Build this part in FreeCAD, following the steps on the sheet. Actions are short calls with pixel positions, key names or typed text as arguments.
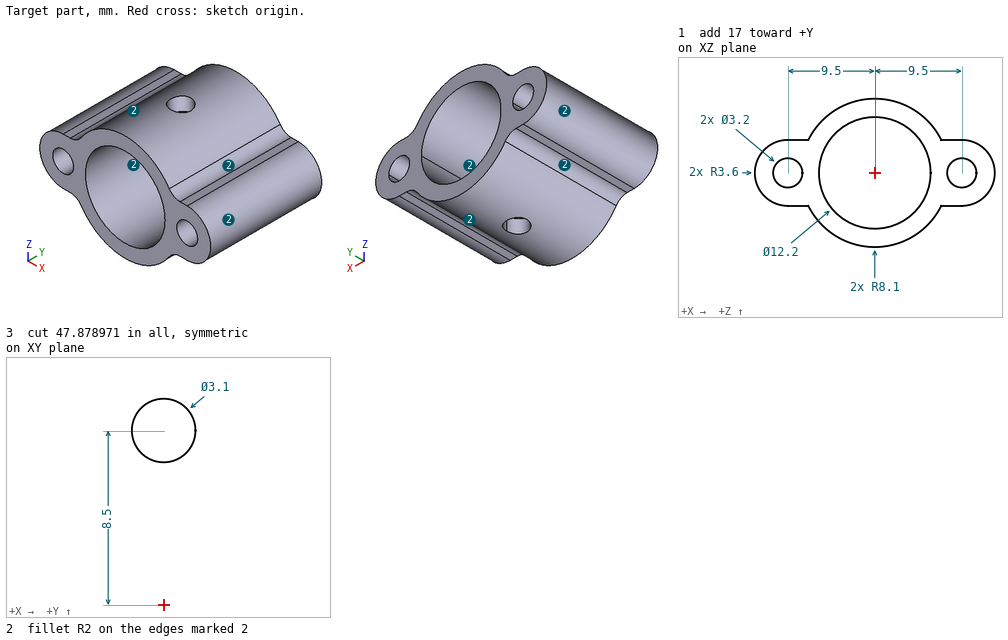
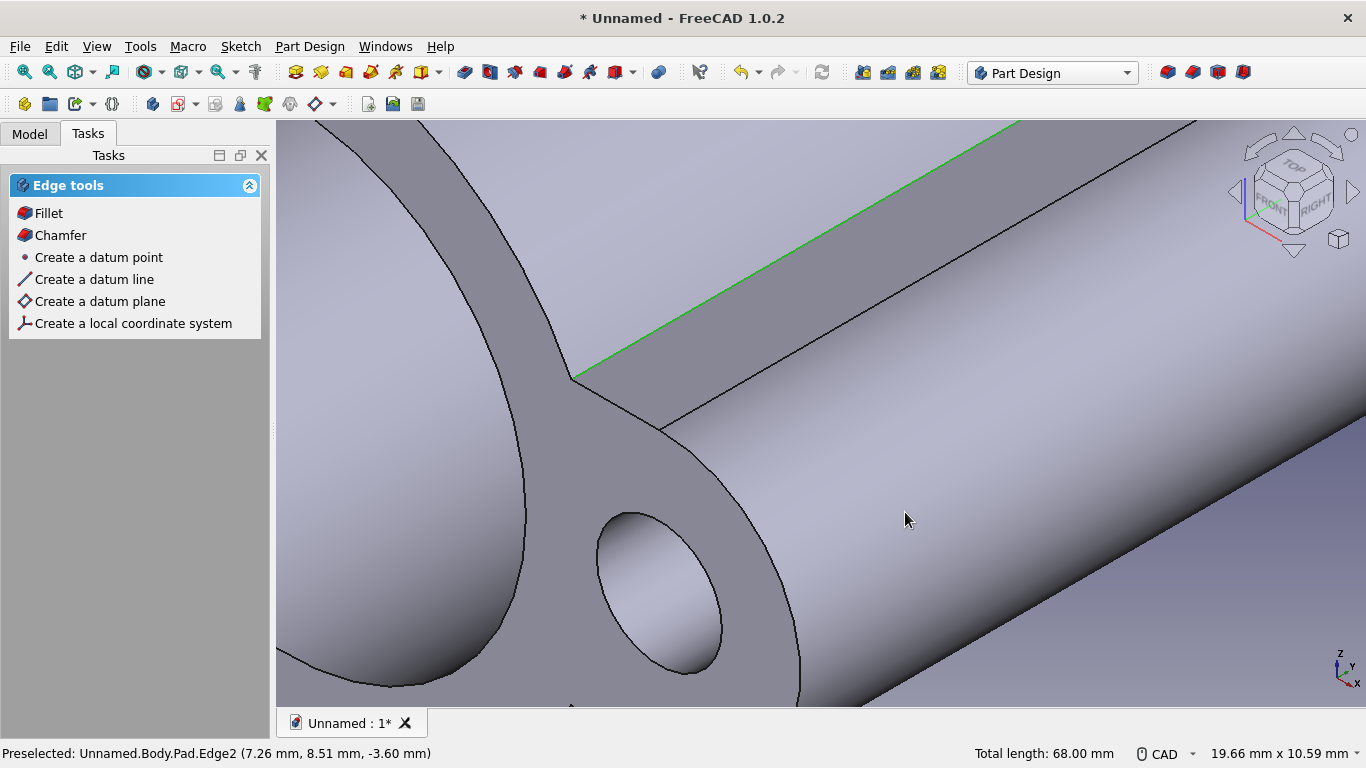
click(1168, 72)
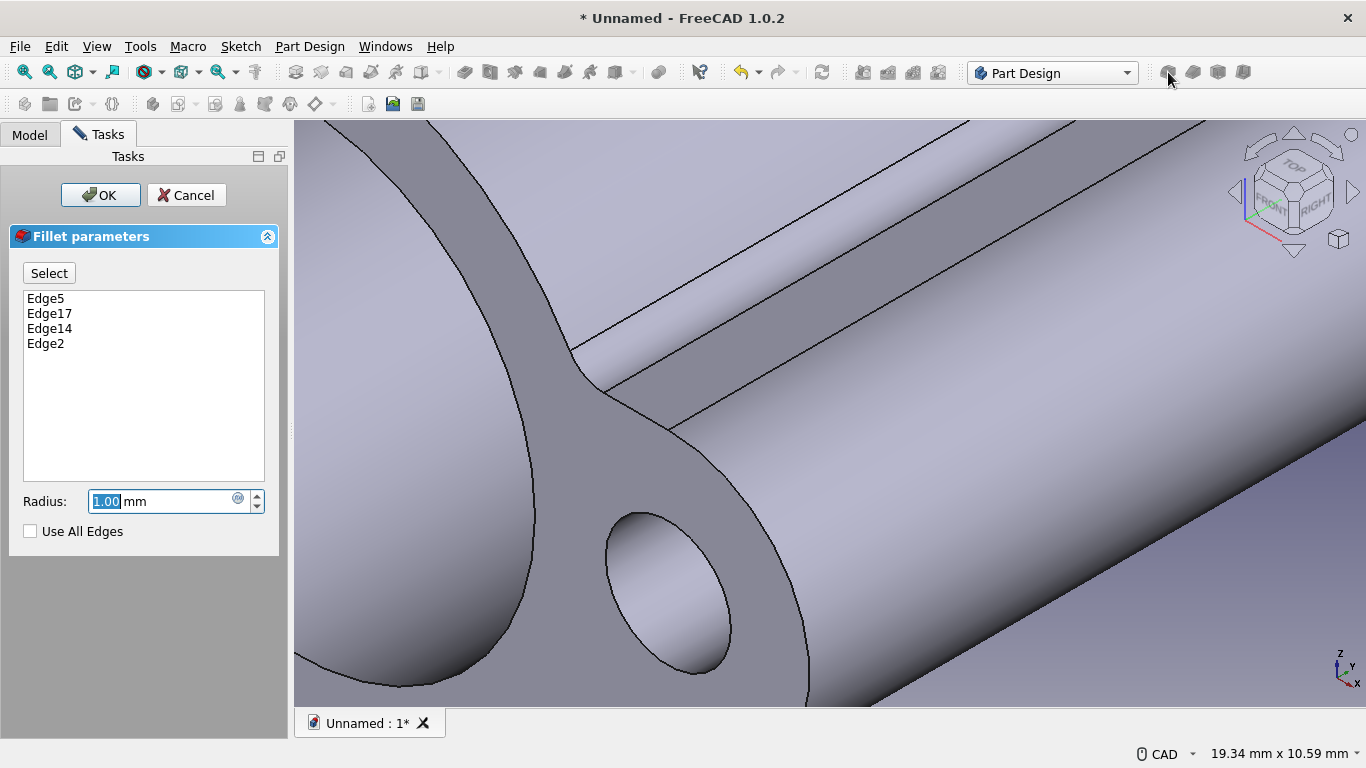
text(2)
key(Tab)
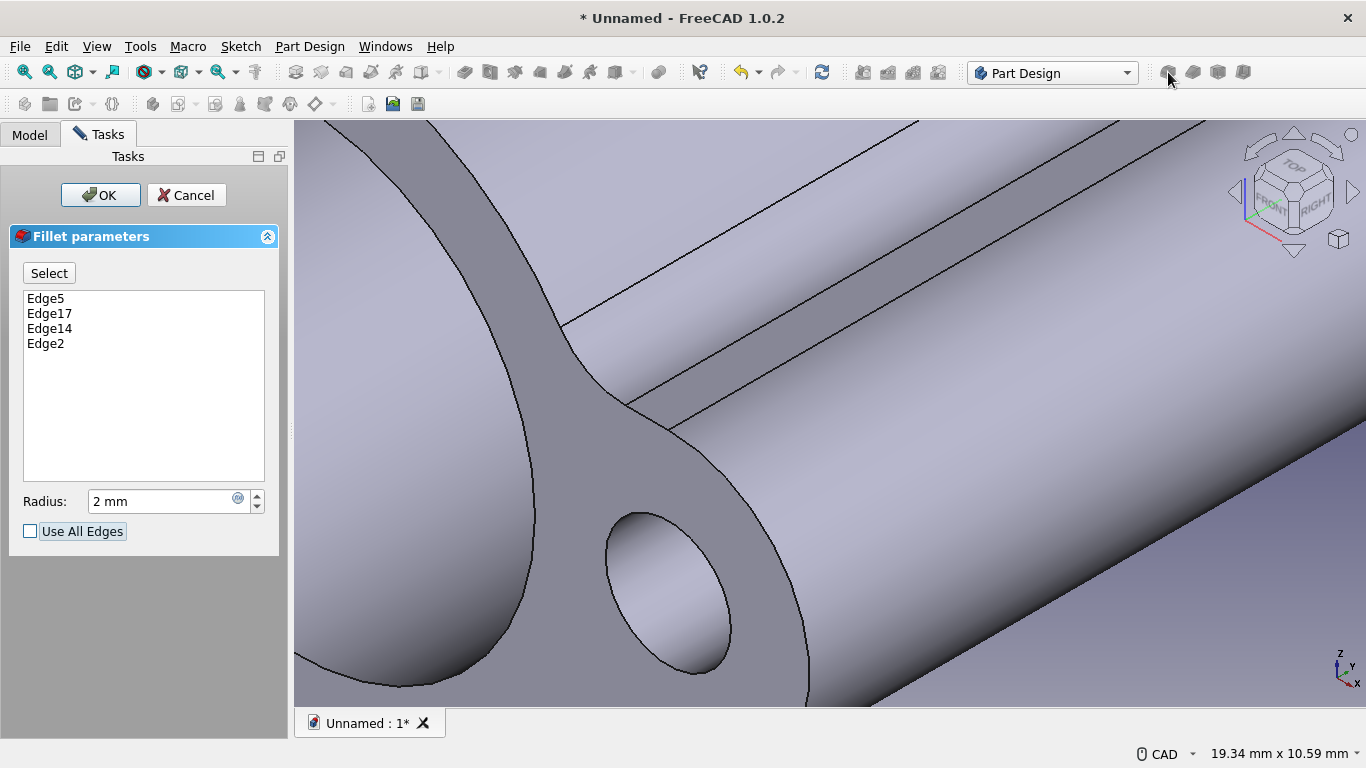
click(101, 195)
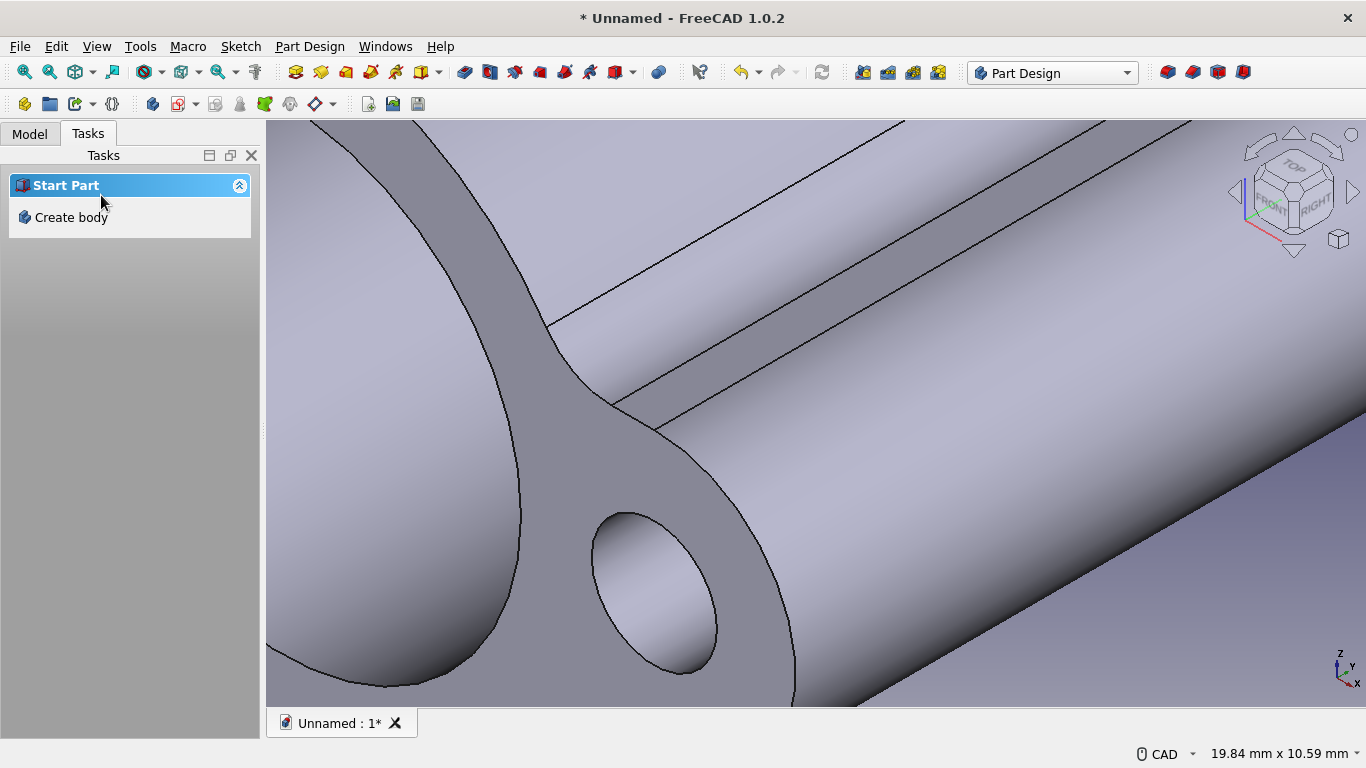
key(v)
key(f)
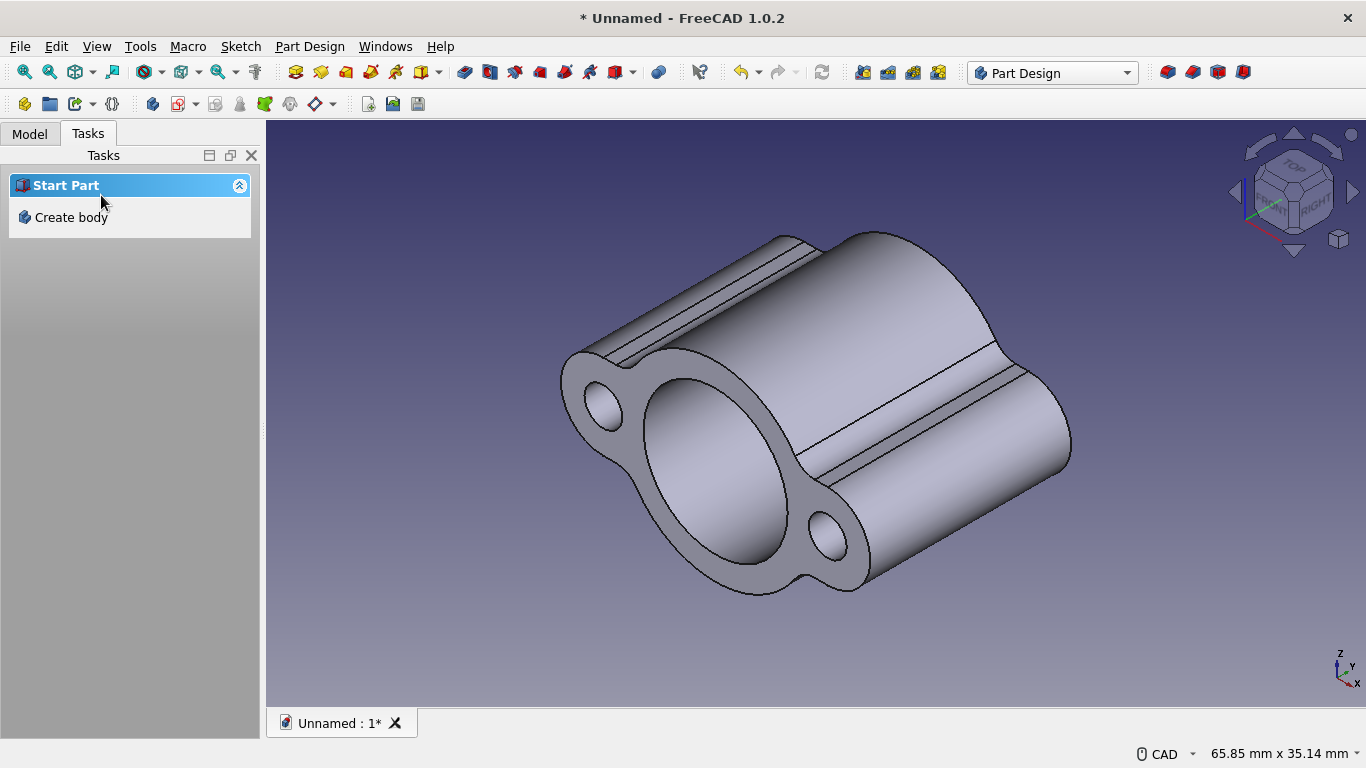
click(178, 104)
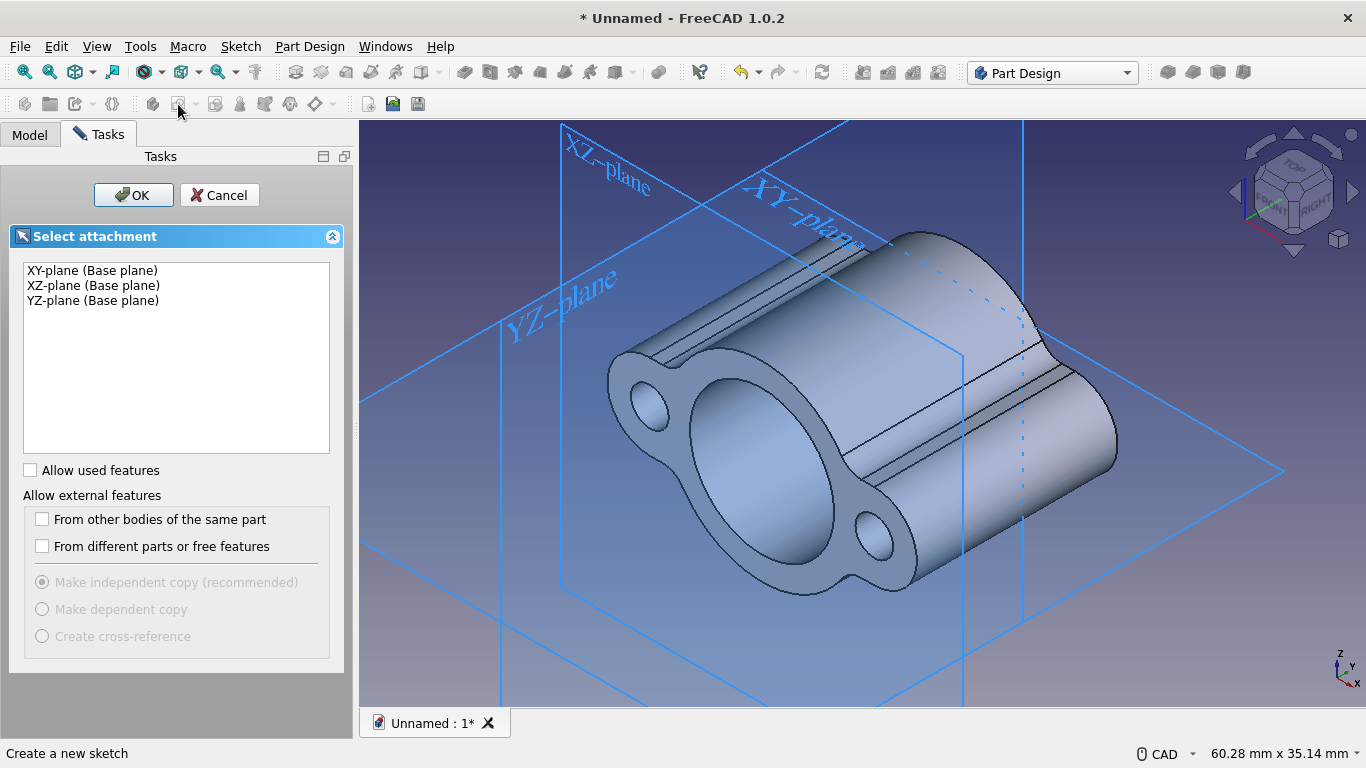
click(84, 270)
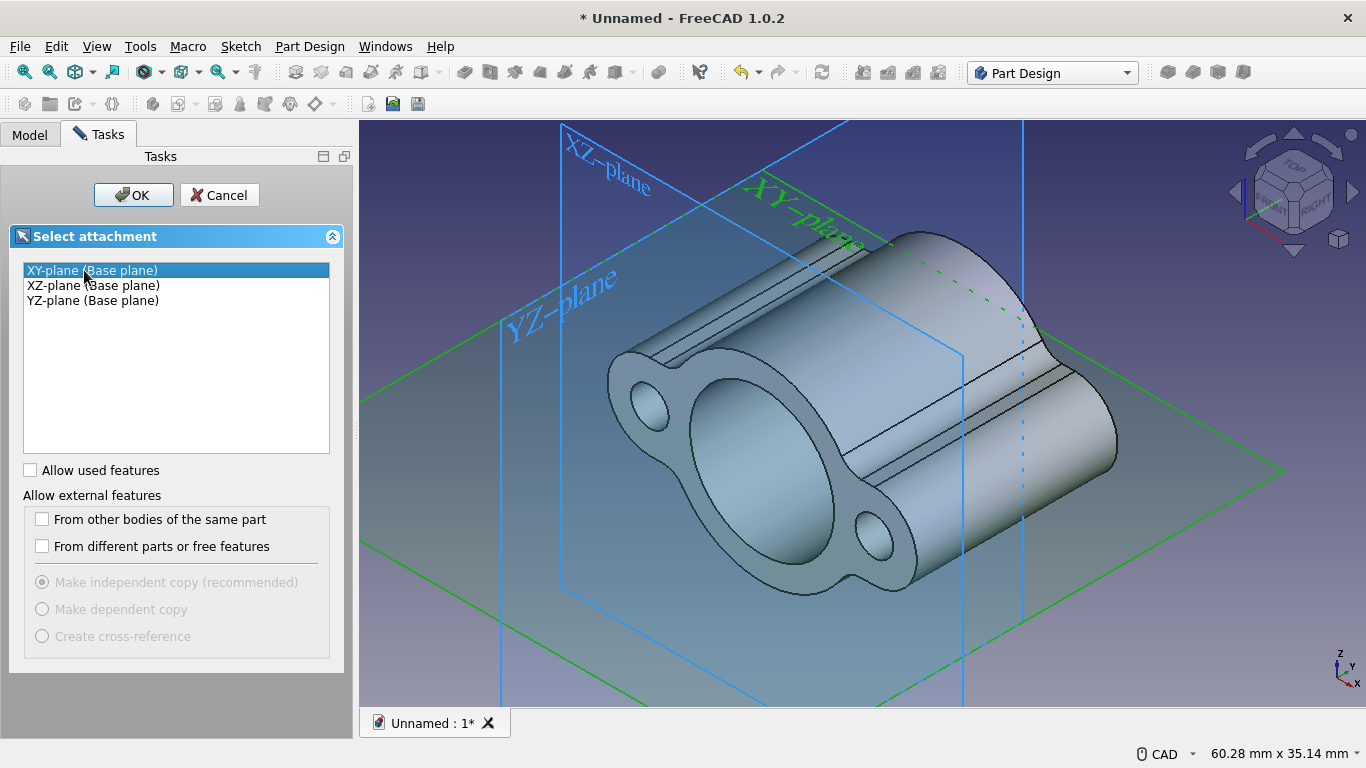
click(134, 195)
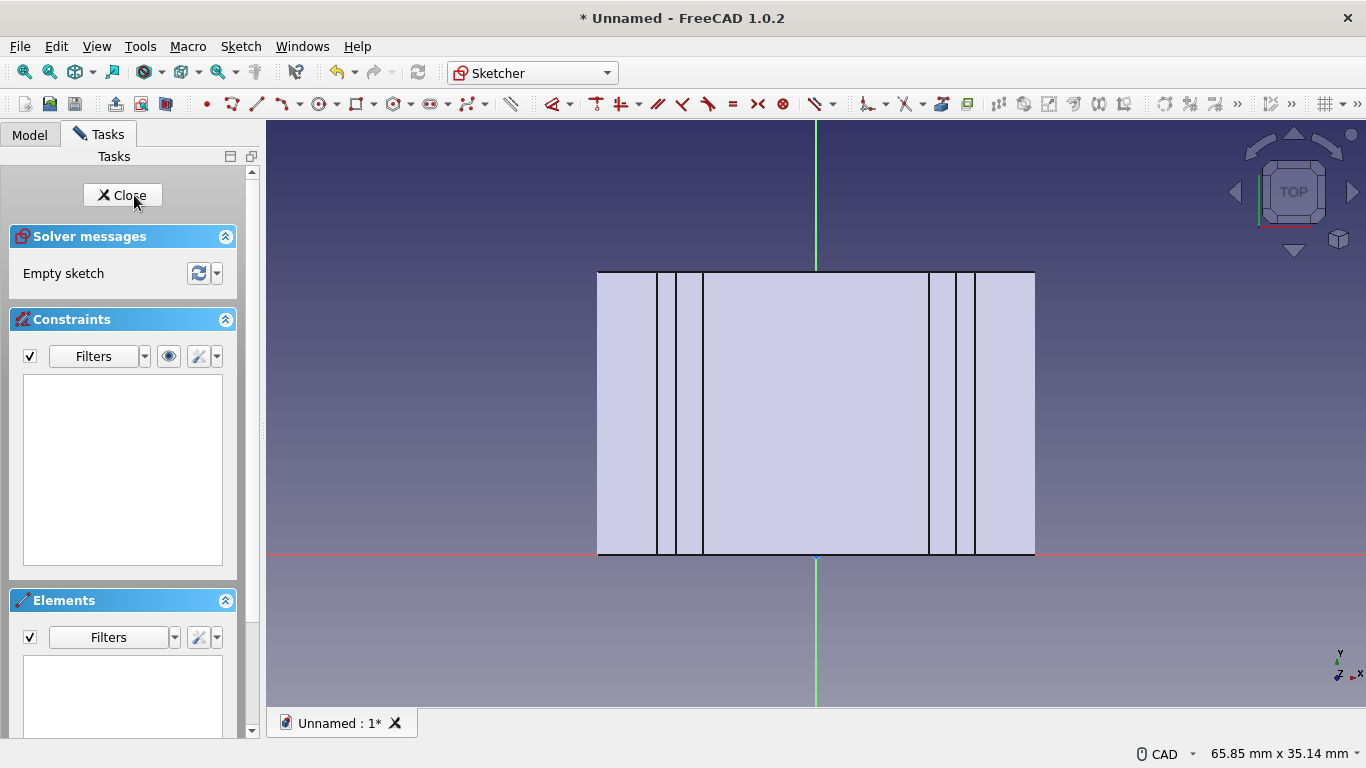
key(q)
key(s)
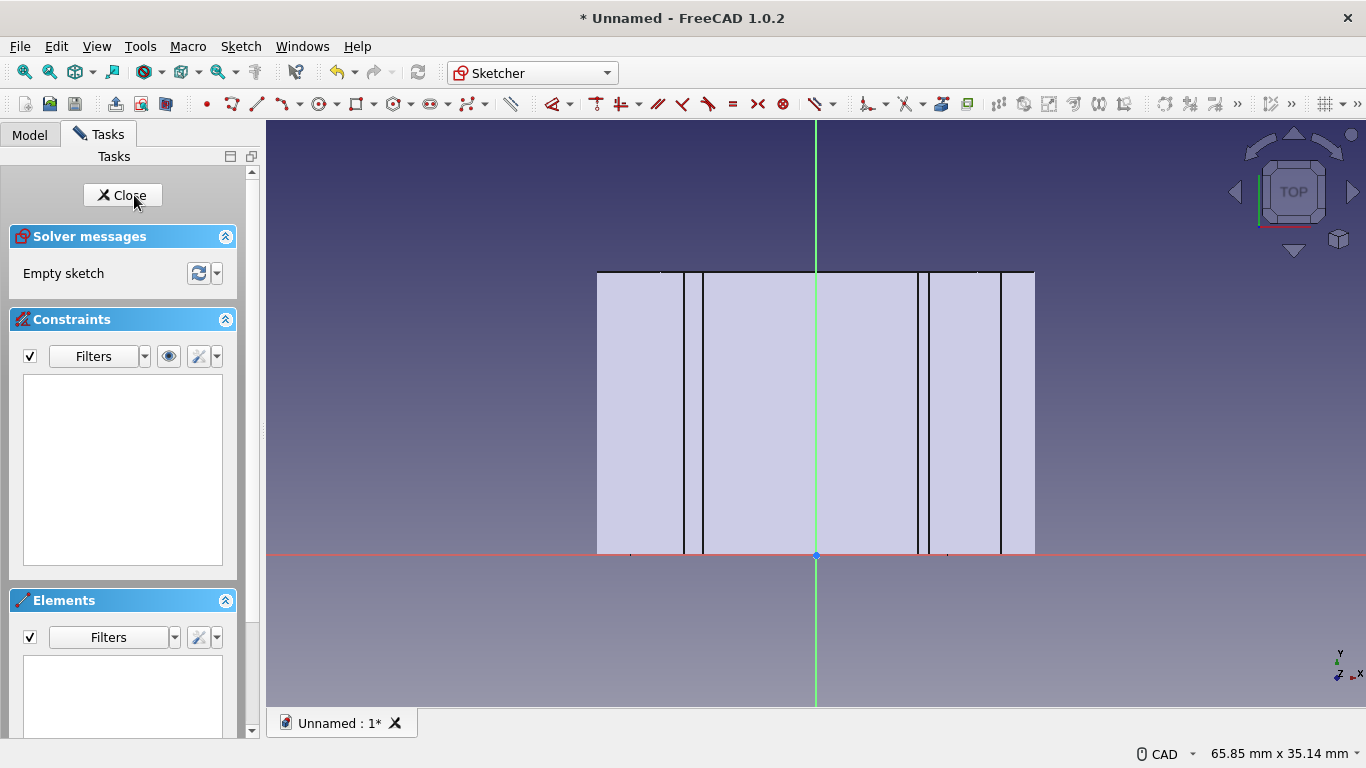
scroll(827, 414, up, 10)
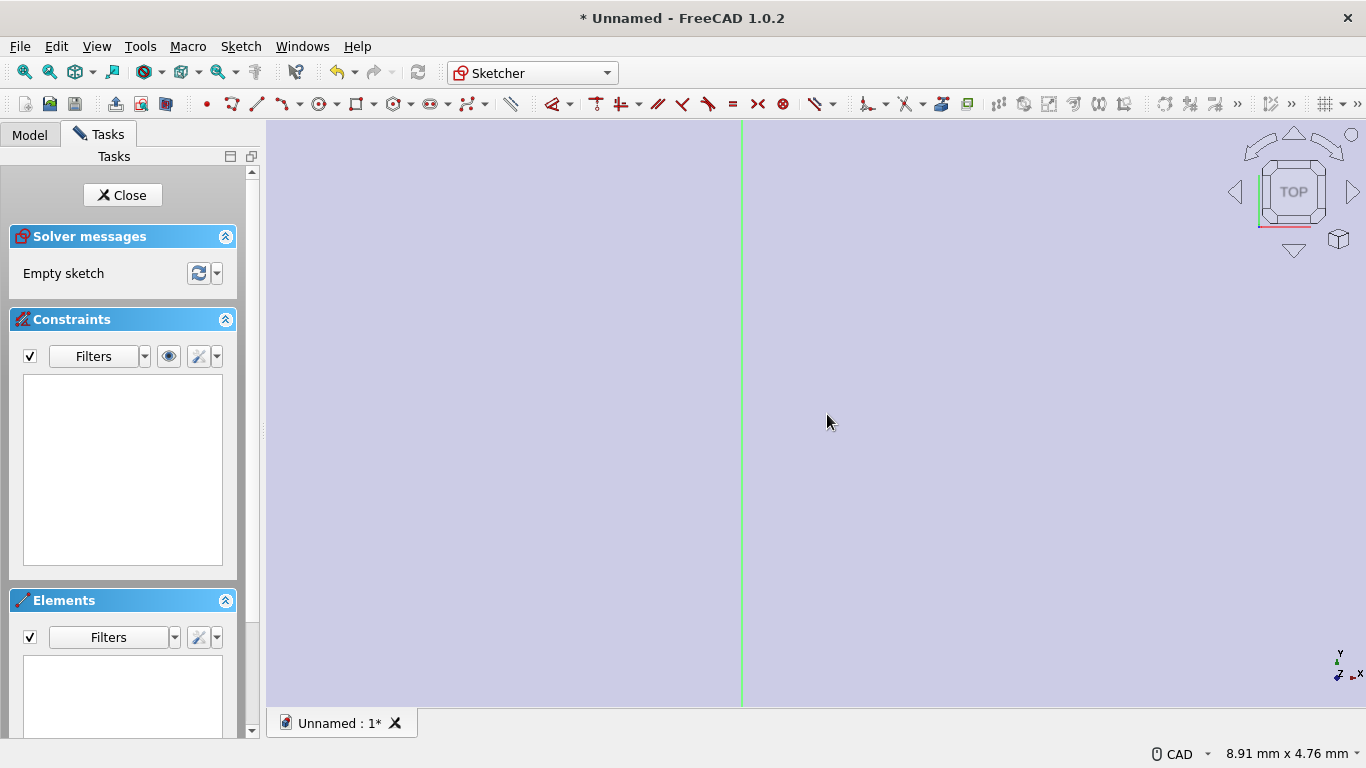
click(318, 104)